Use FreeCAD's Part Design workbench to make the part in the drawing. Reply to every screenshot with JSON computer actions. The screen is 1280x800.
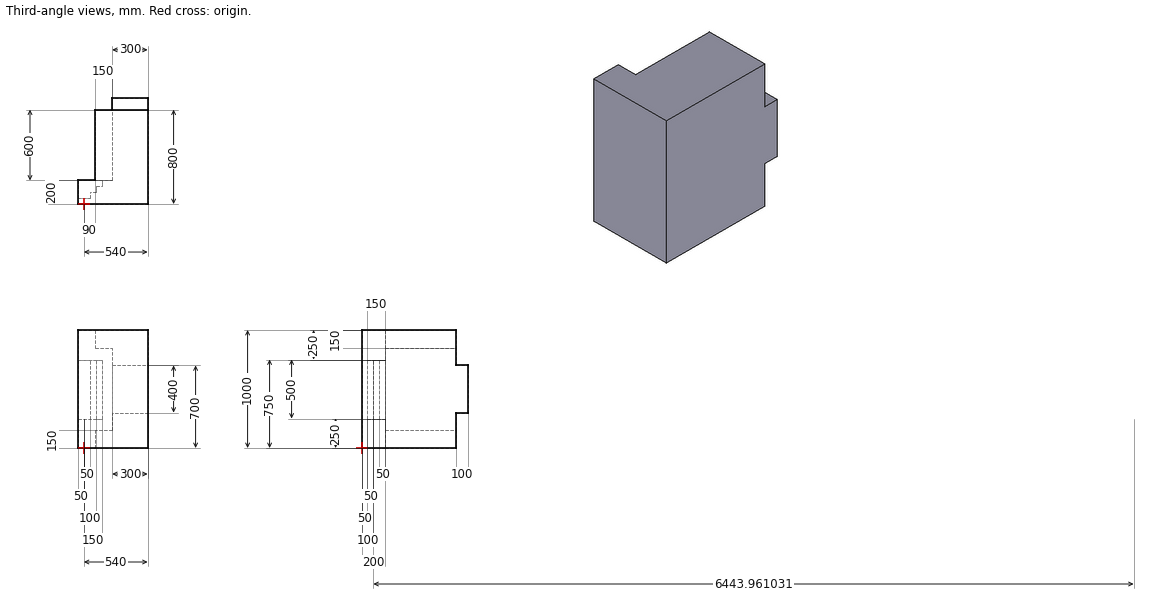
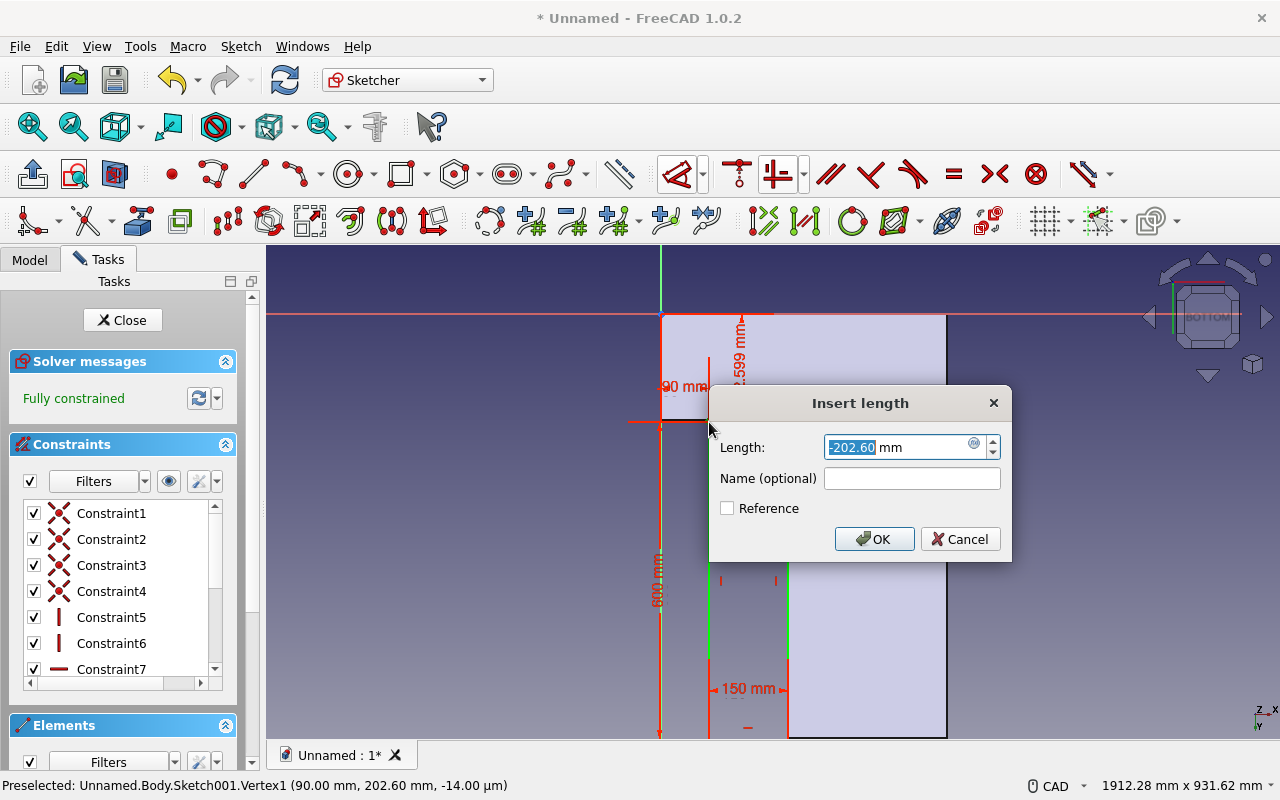
{"action": "type", "text": "-200"}
{"action": "key", "text": "Return"}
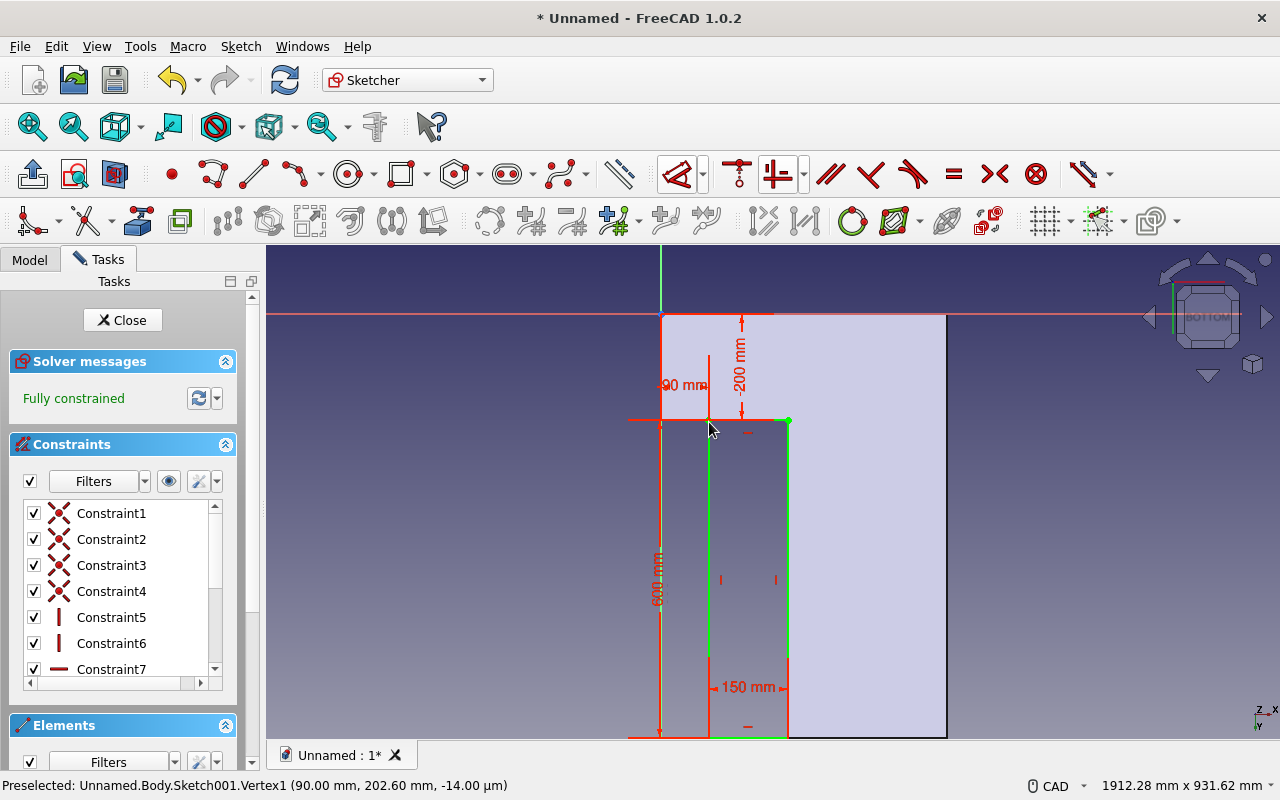
{"action": "left_click", "coordinate": [123, 320]}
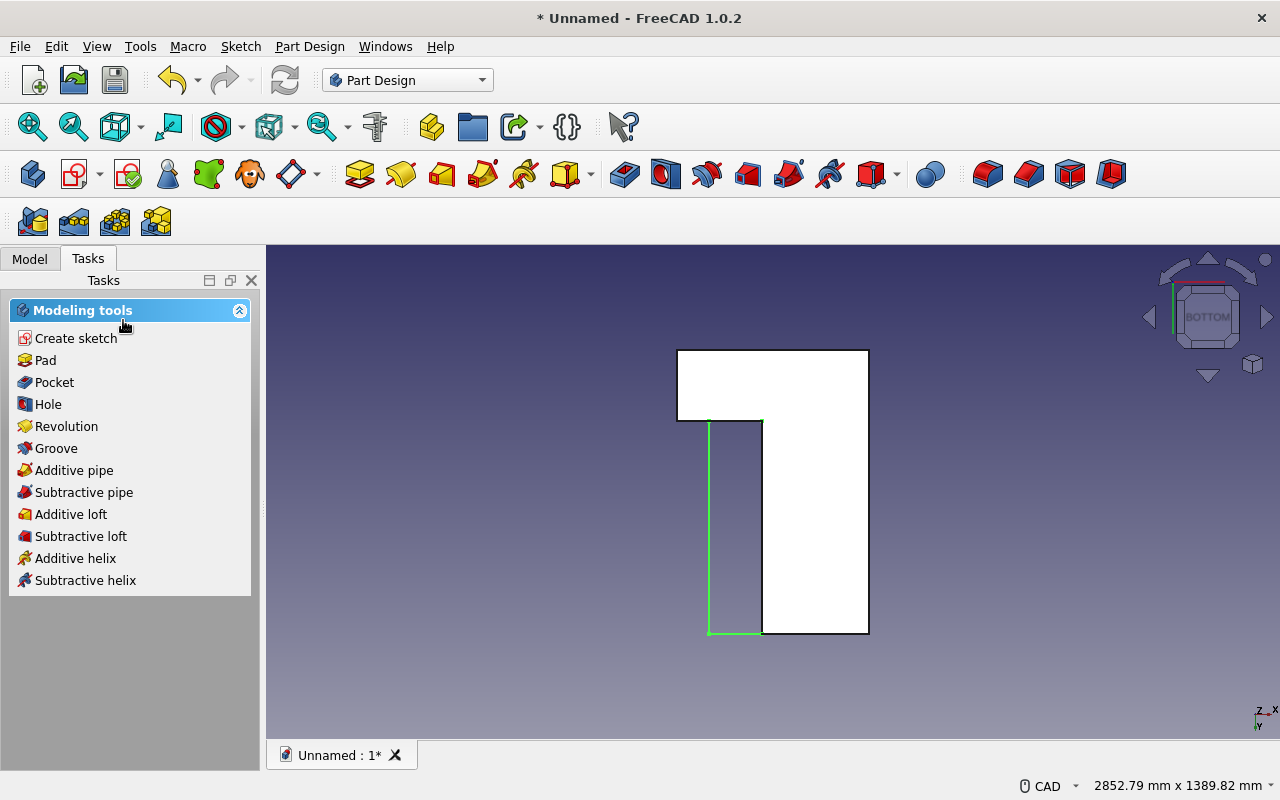
{"action": "left_click", "coordinate": [360, 174]}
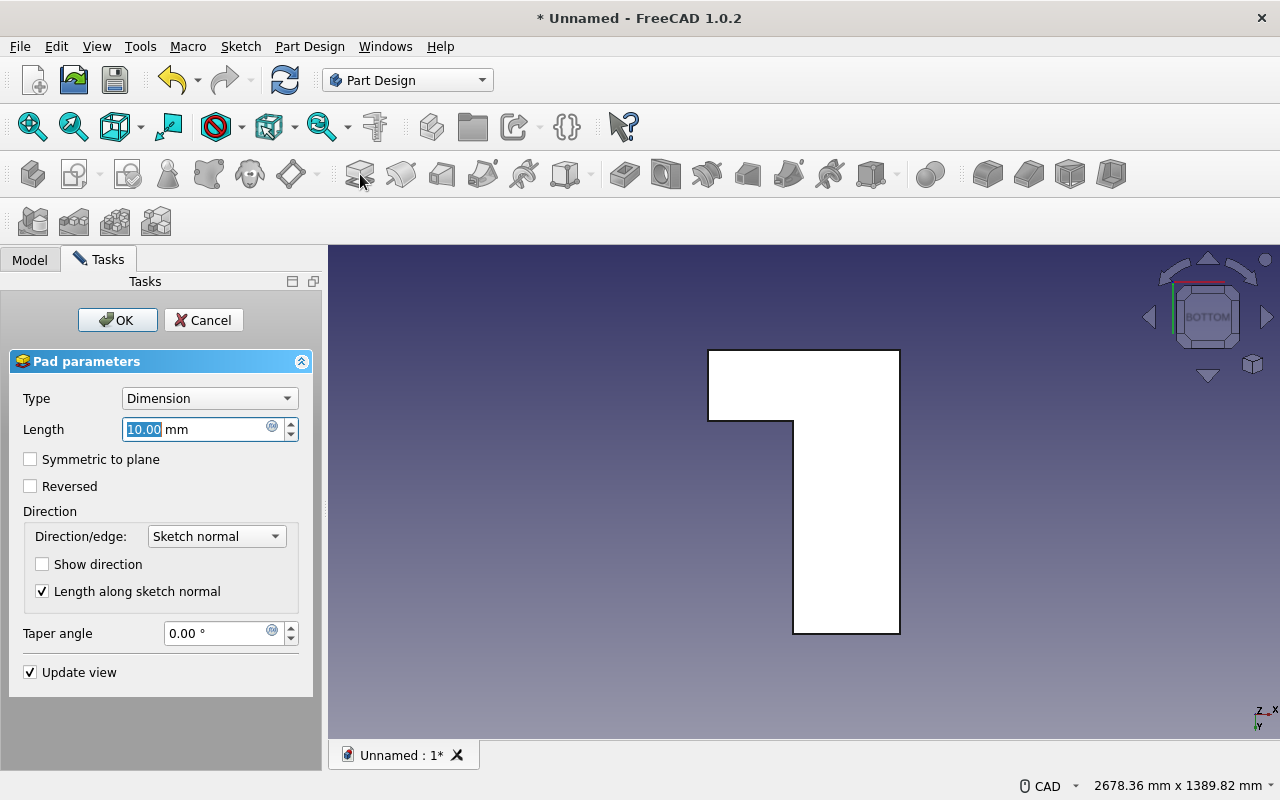
{"action": "type", "text": "150"}
{"action": "key", "text": "Tab"}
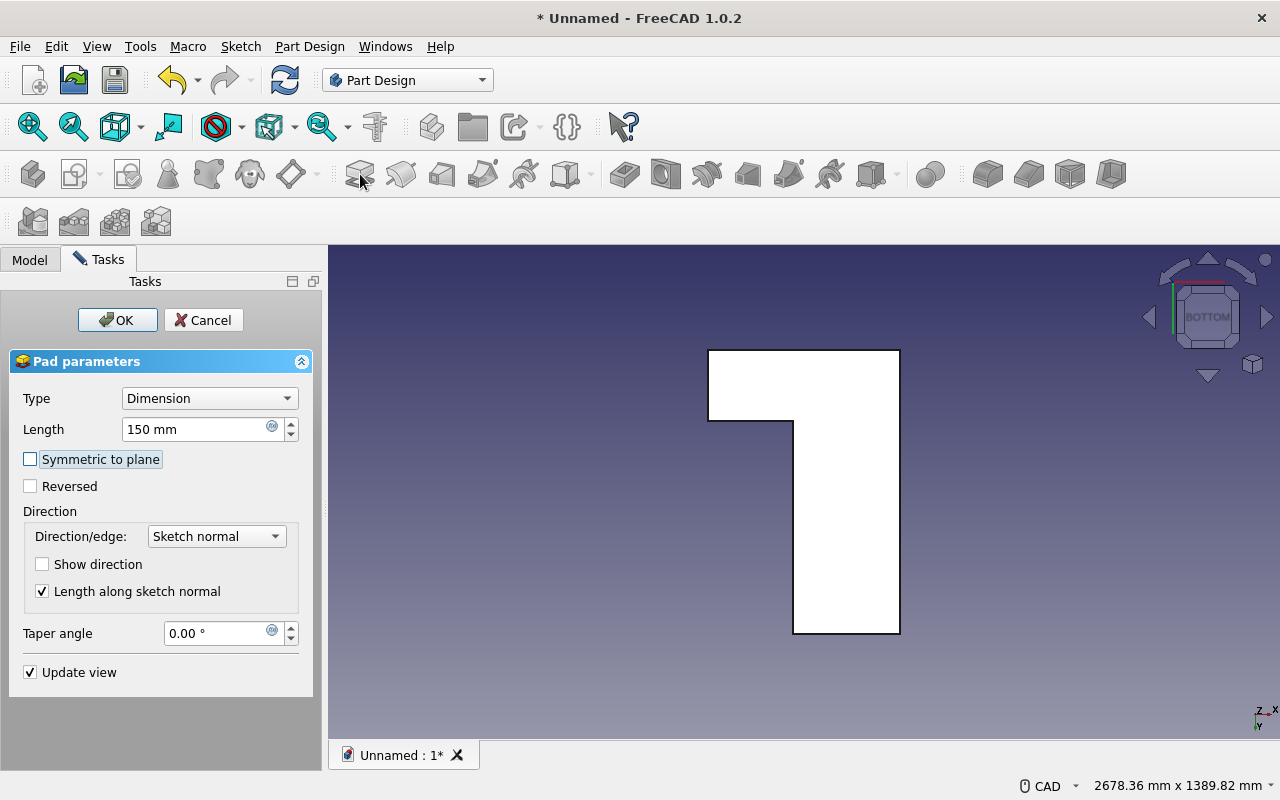
{"action": "left_click", "coordinate": [31, 486]}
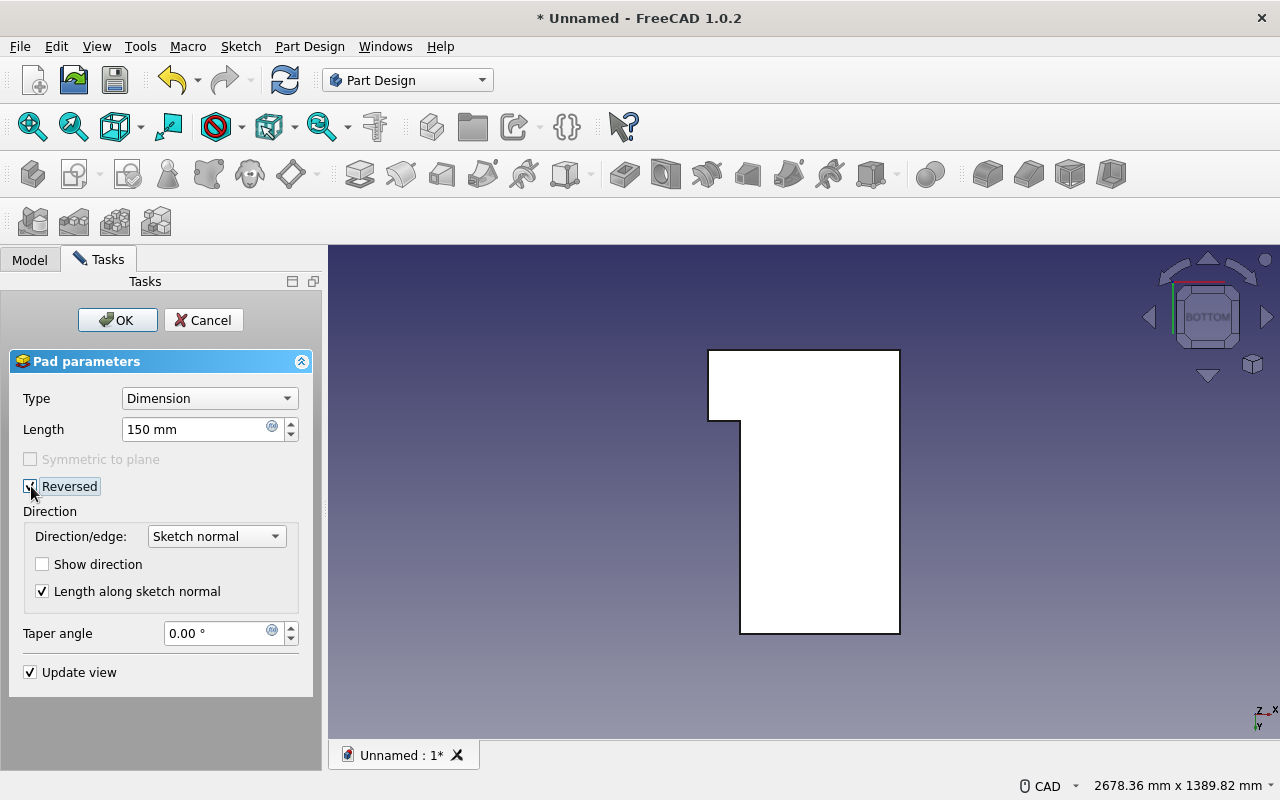
{"action": "left_click", "coordinate": [118, 320]}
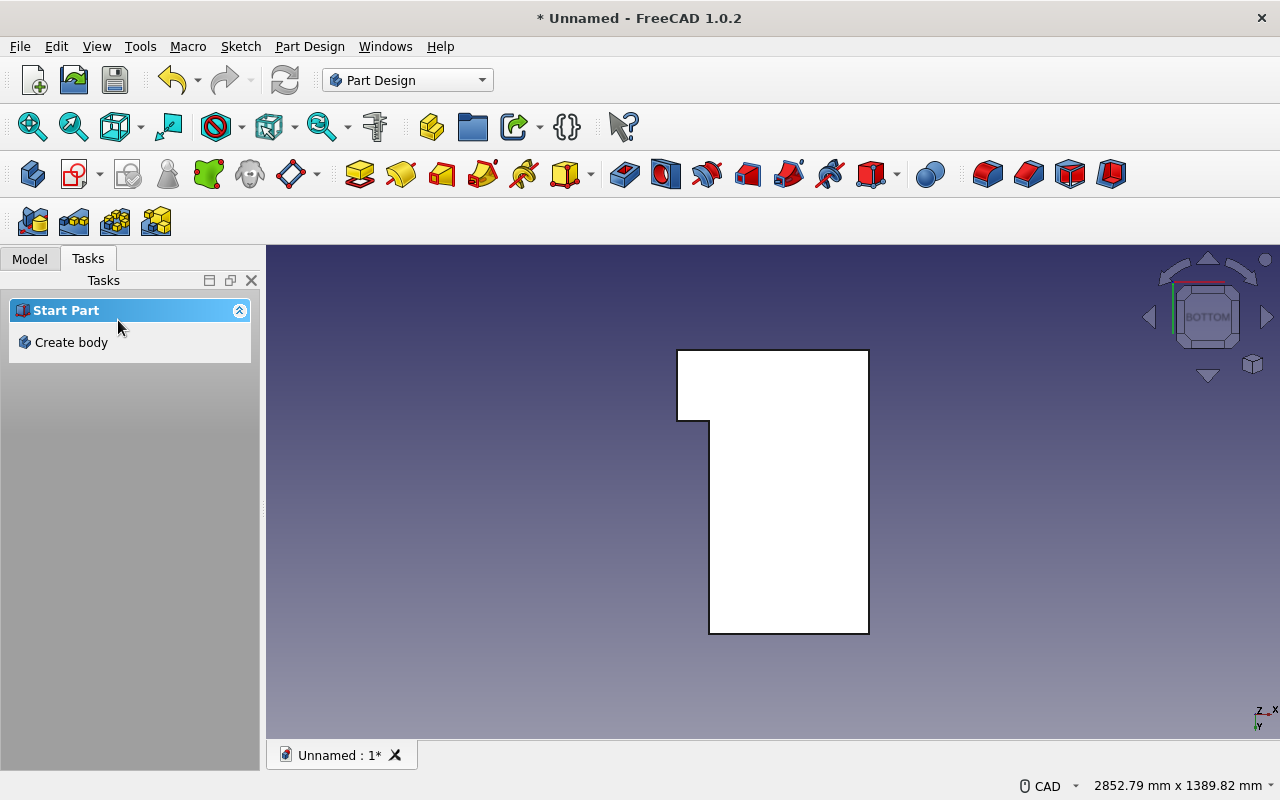
{"action": "key", "text": "0"}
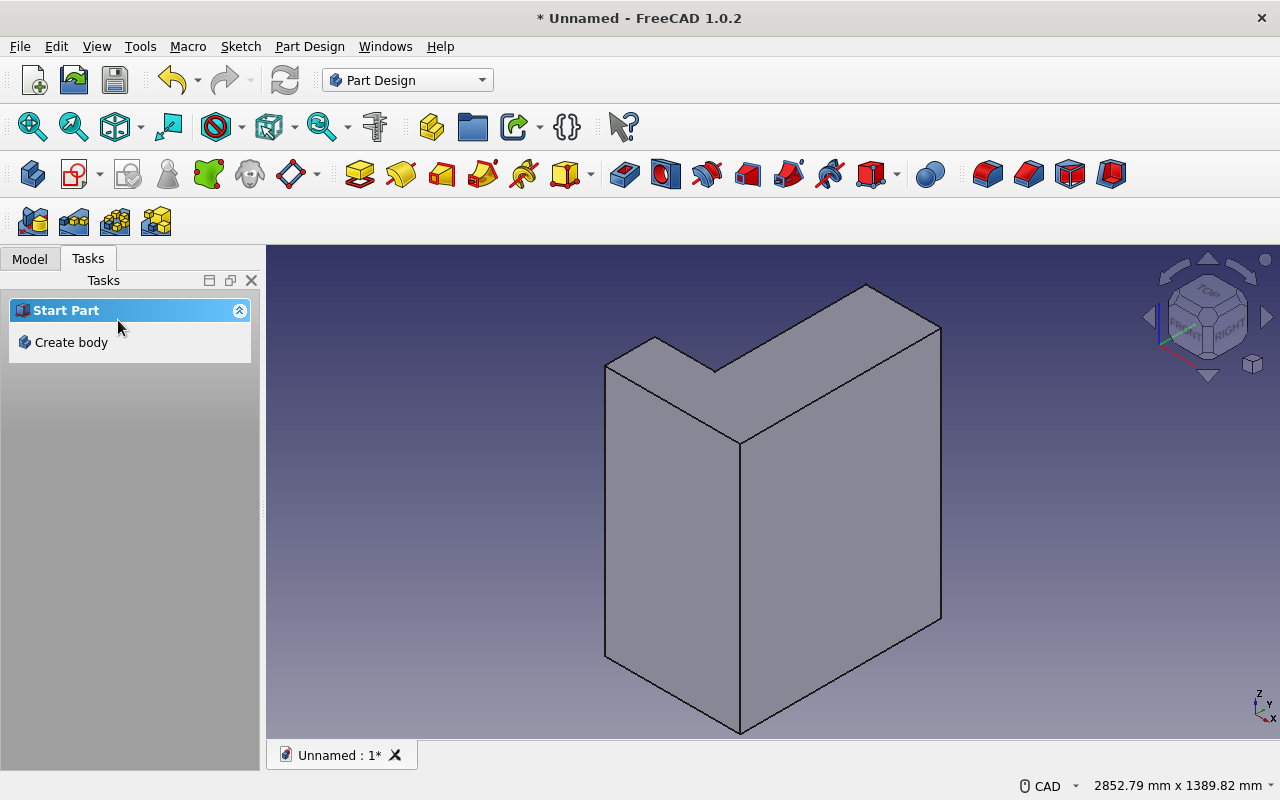
{"action": "left_click", "coordinate": [869, 335]}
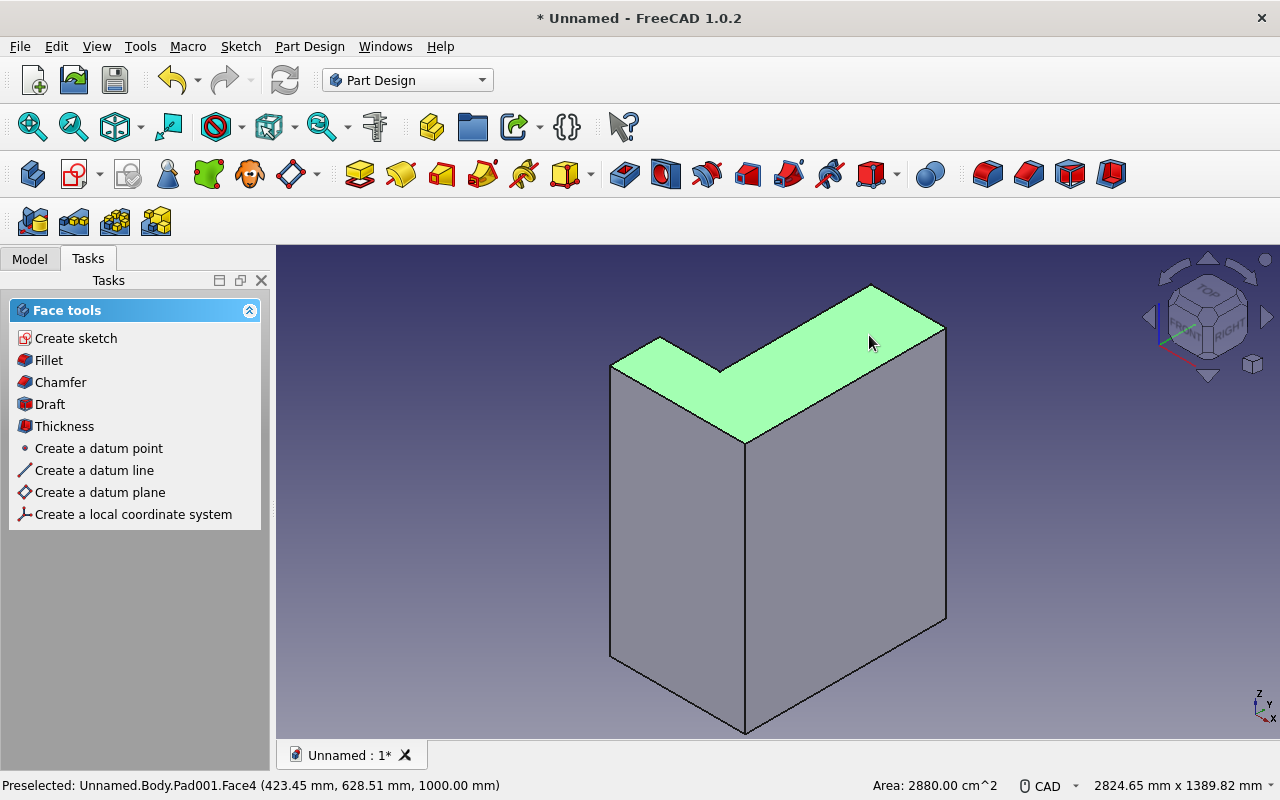
{"action": "left_click", "coordinate": [74, 174]}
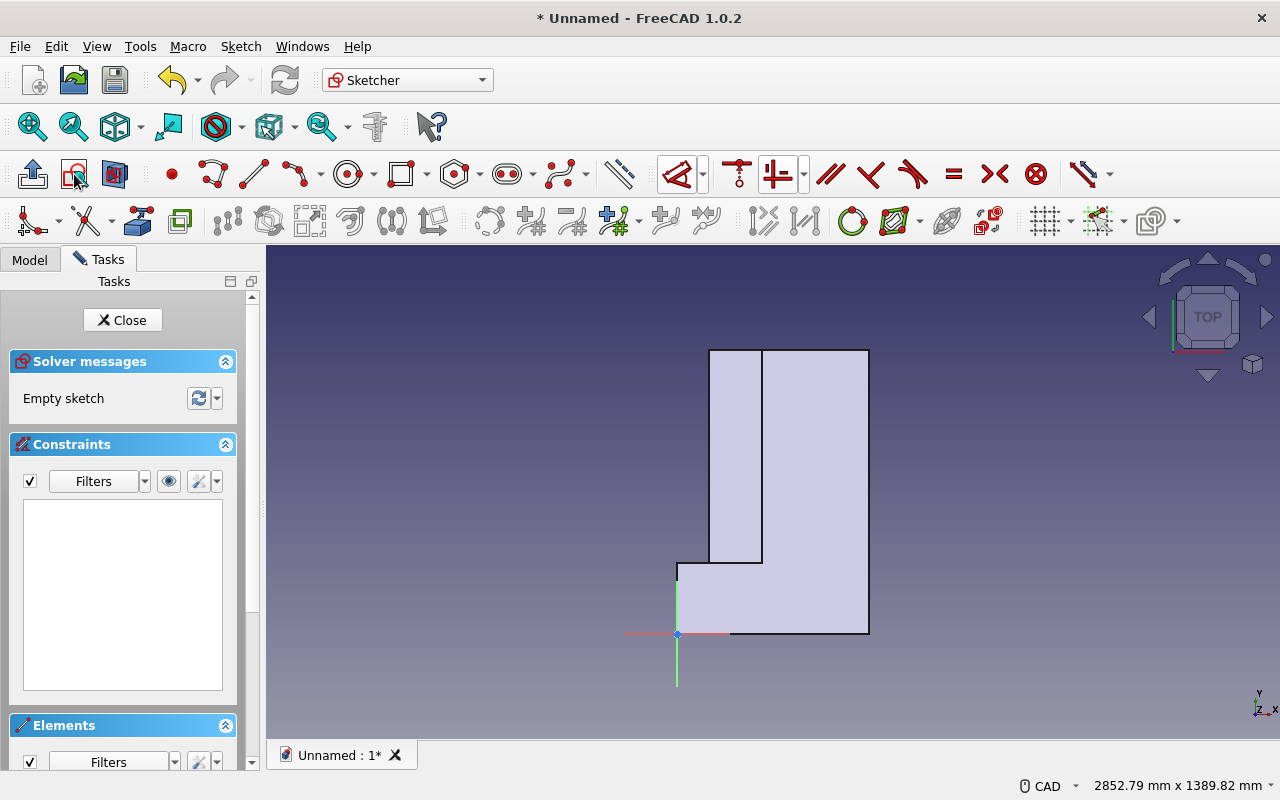
{"action": "left_click", "coordinate": [400, 174]}